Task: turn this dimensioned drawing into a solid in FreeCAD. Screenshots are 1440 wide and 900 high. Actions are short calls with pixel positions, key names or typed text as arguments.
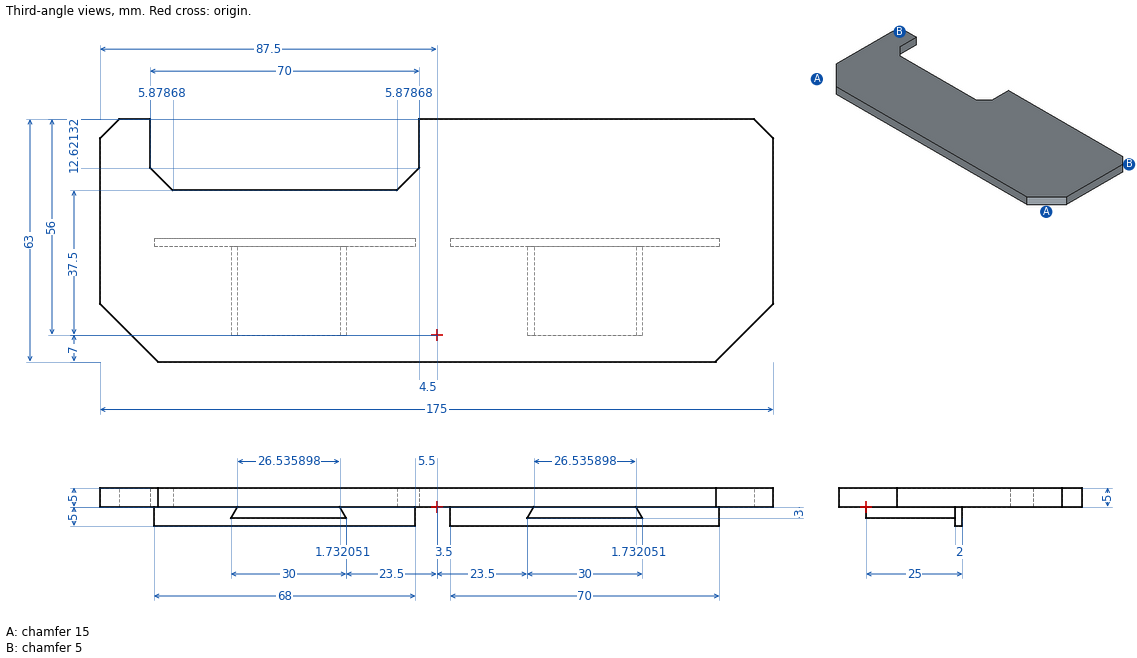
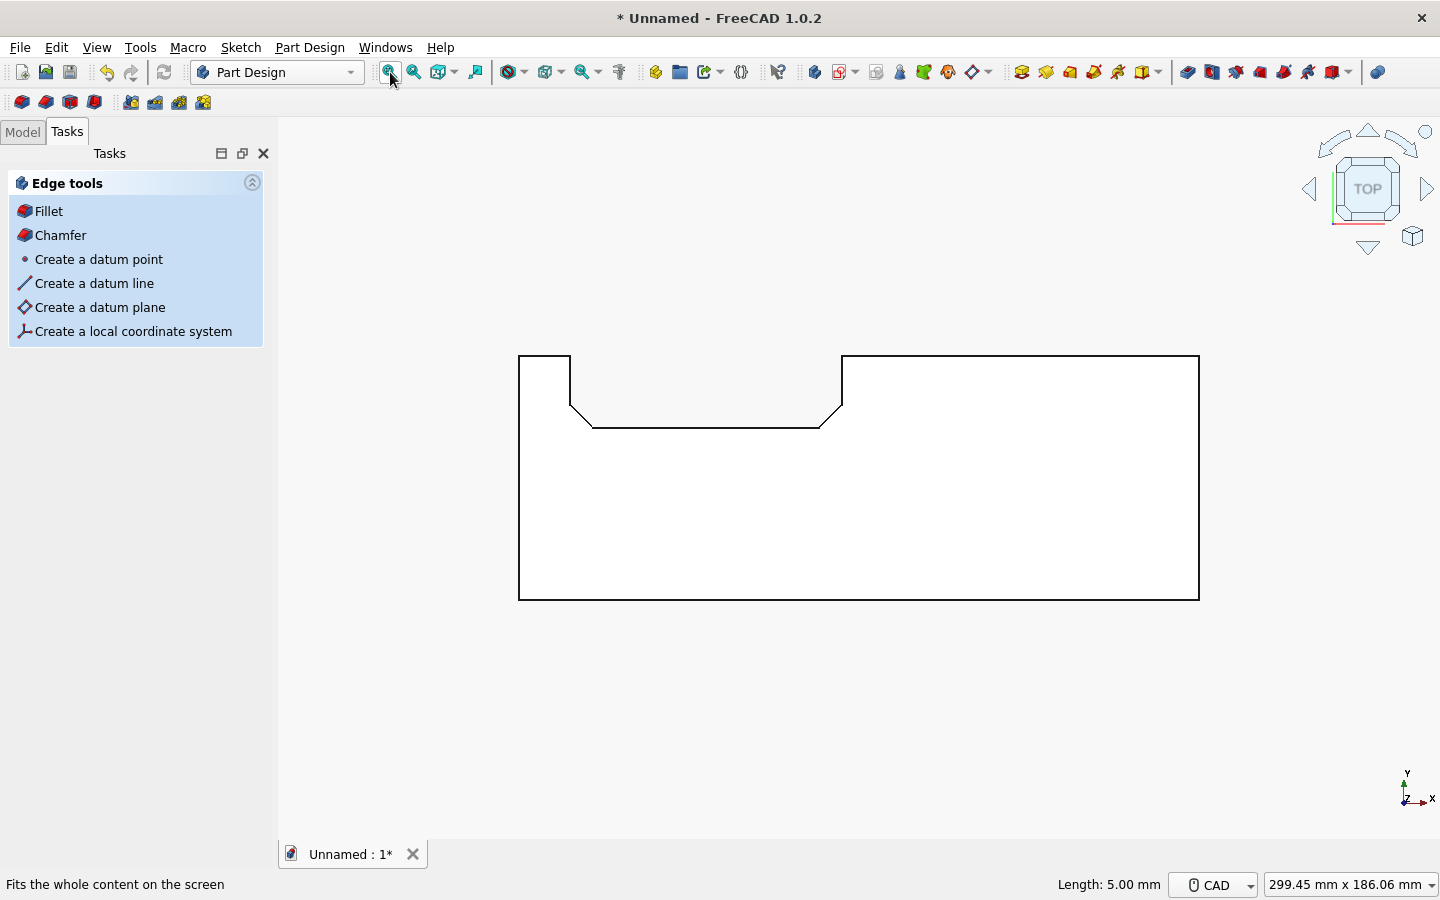
scroll(519, 599, up, 4)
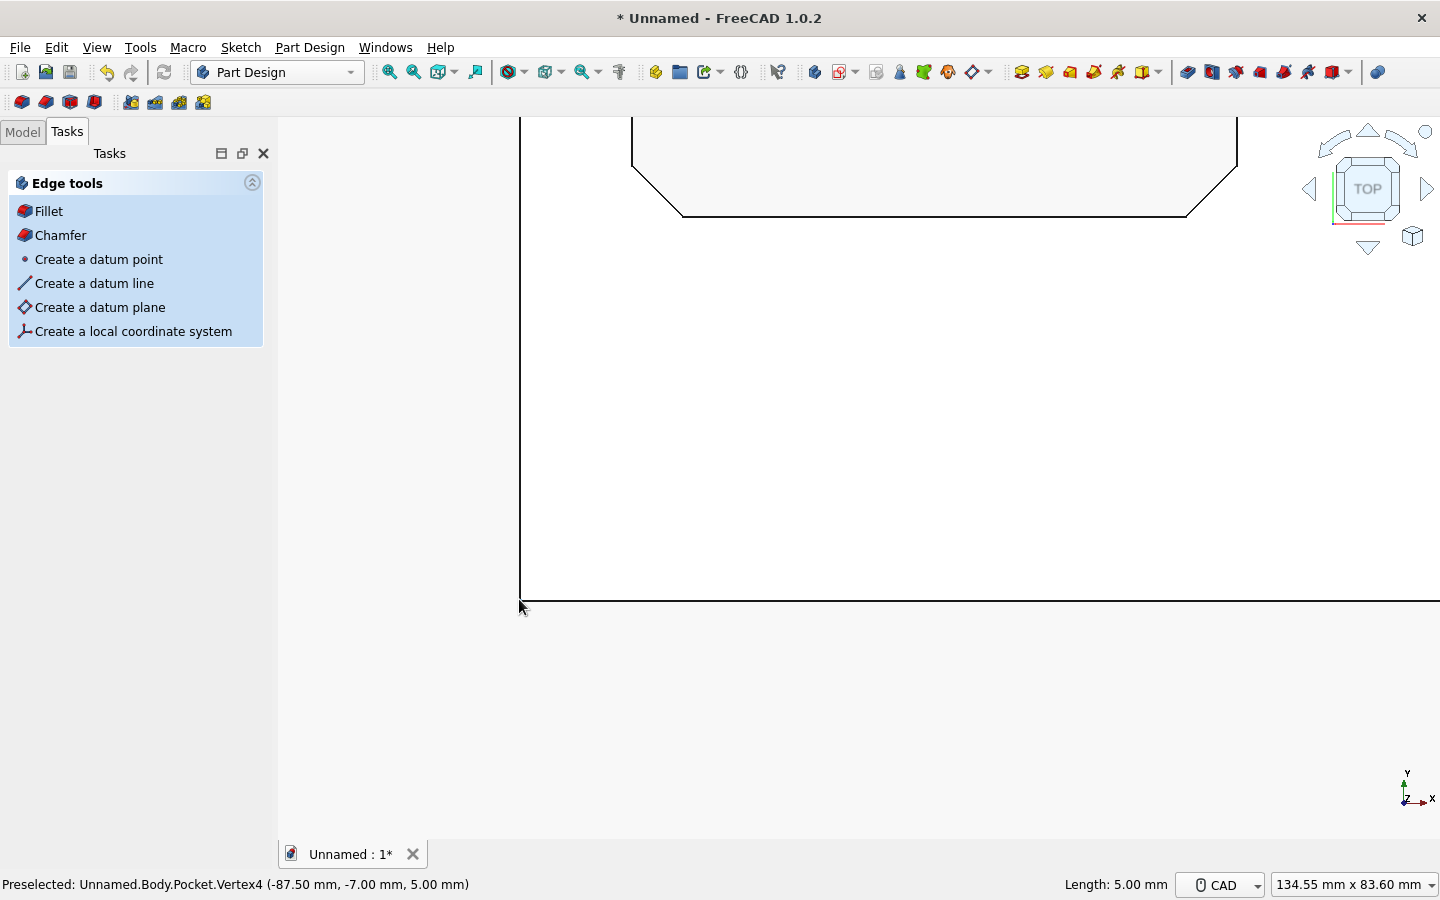
key(v)
key(f)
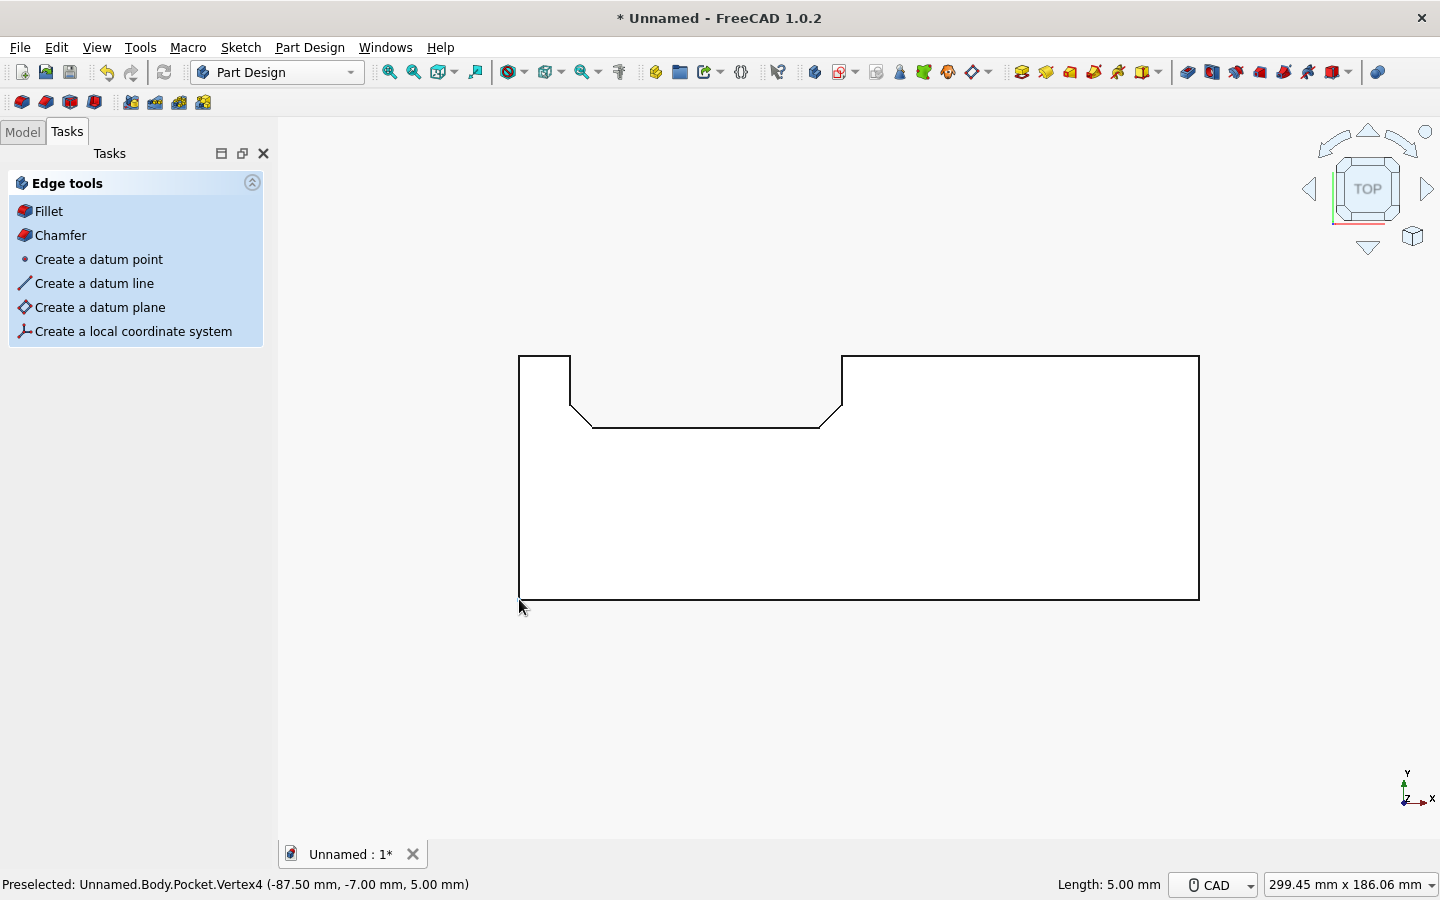
key(1)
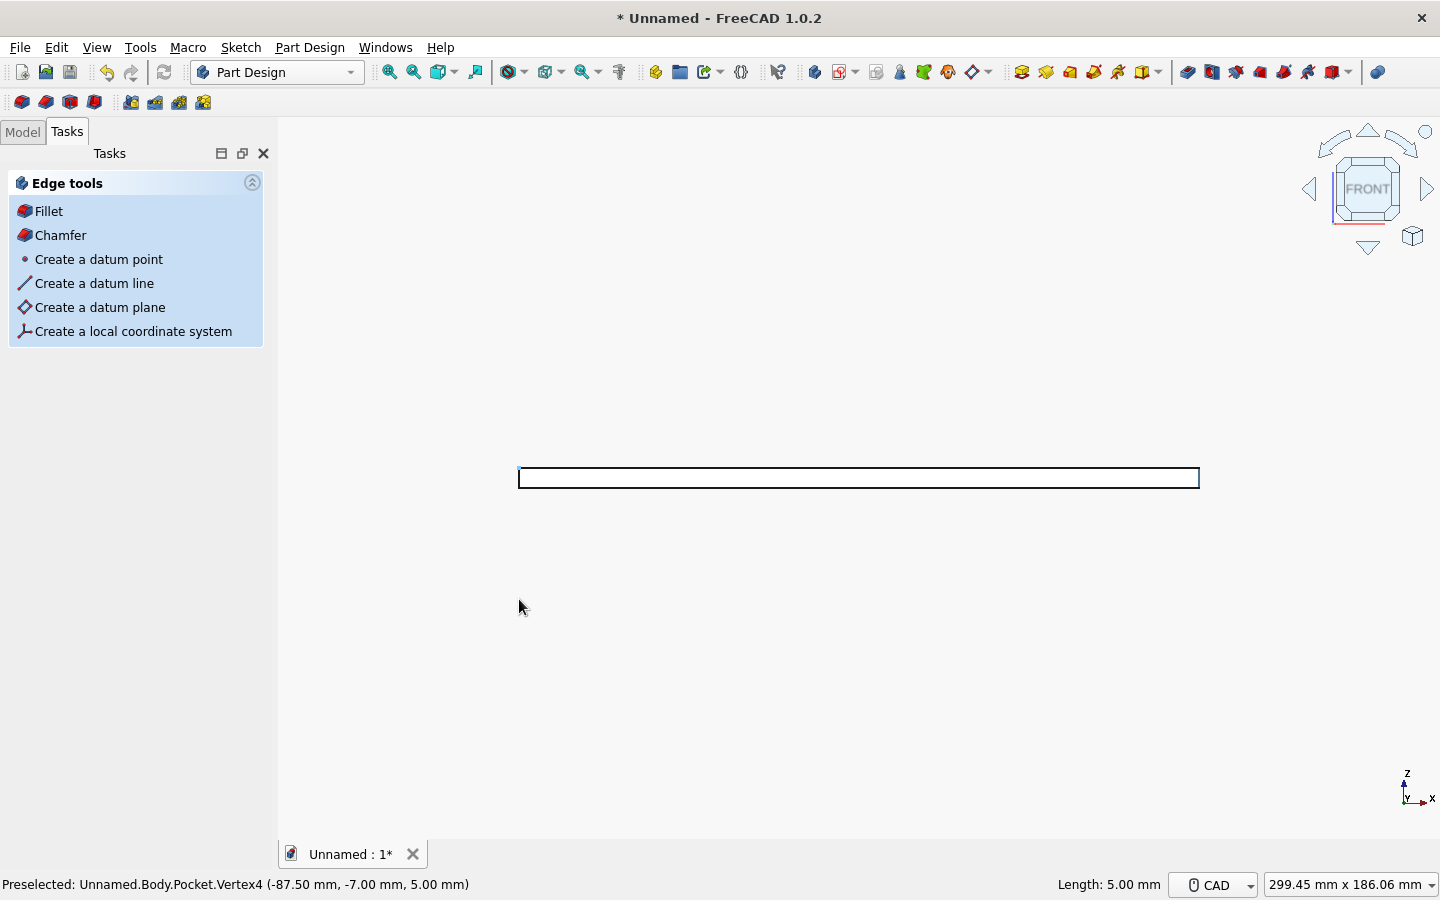
click(519, 477, ctrl)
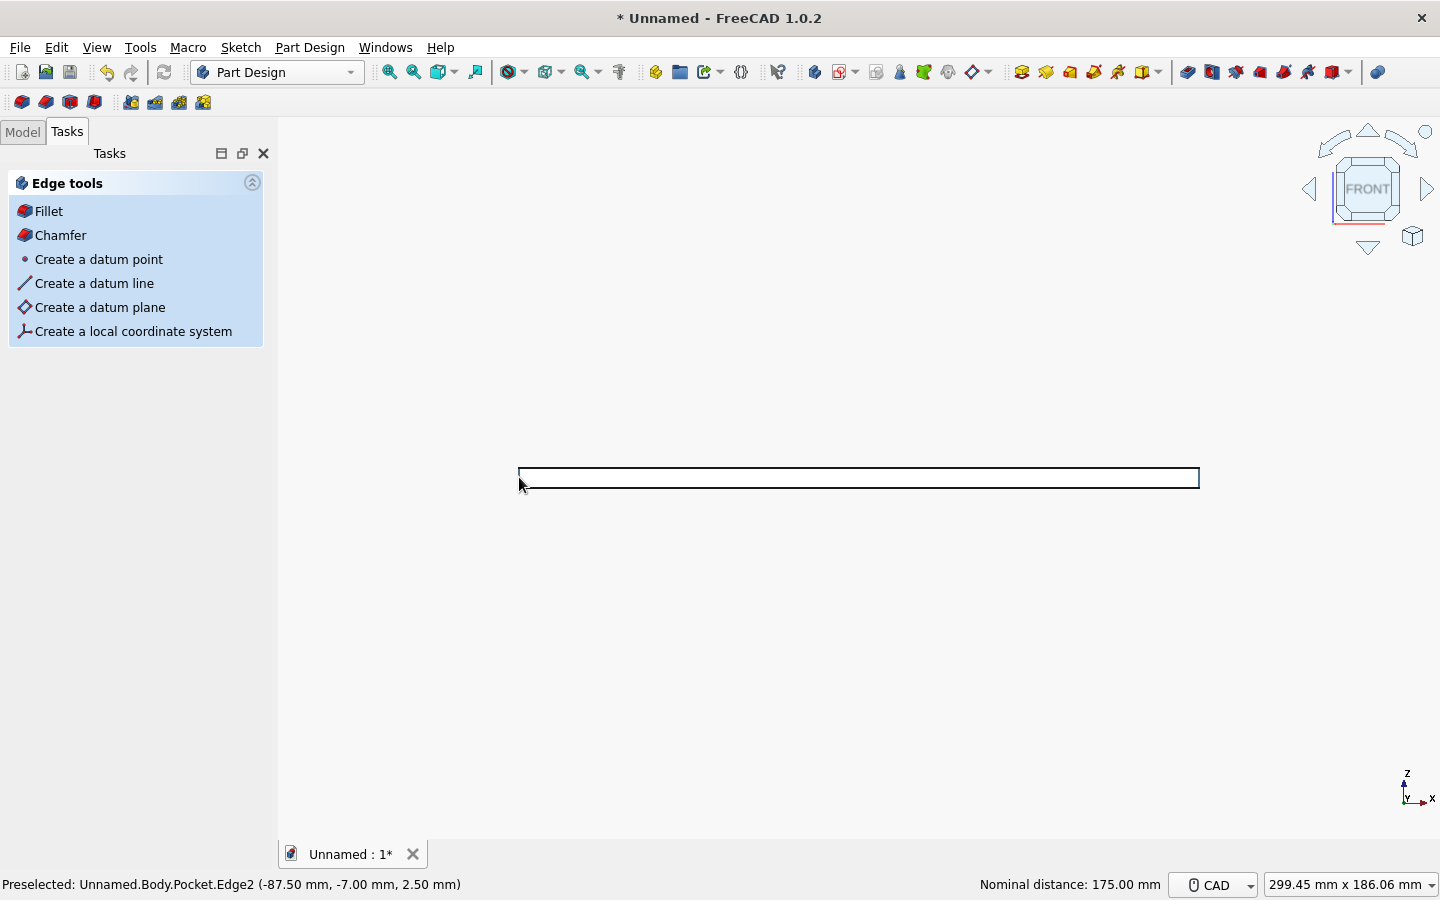
click(46, 102)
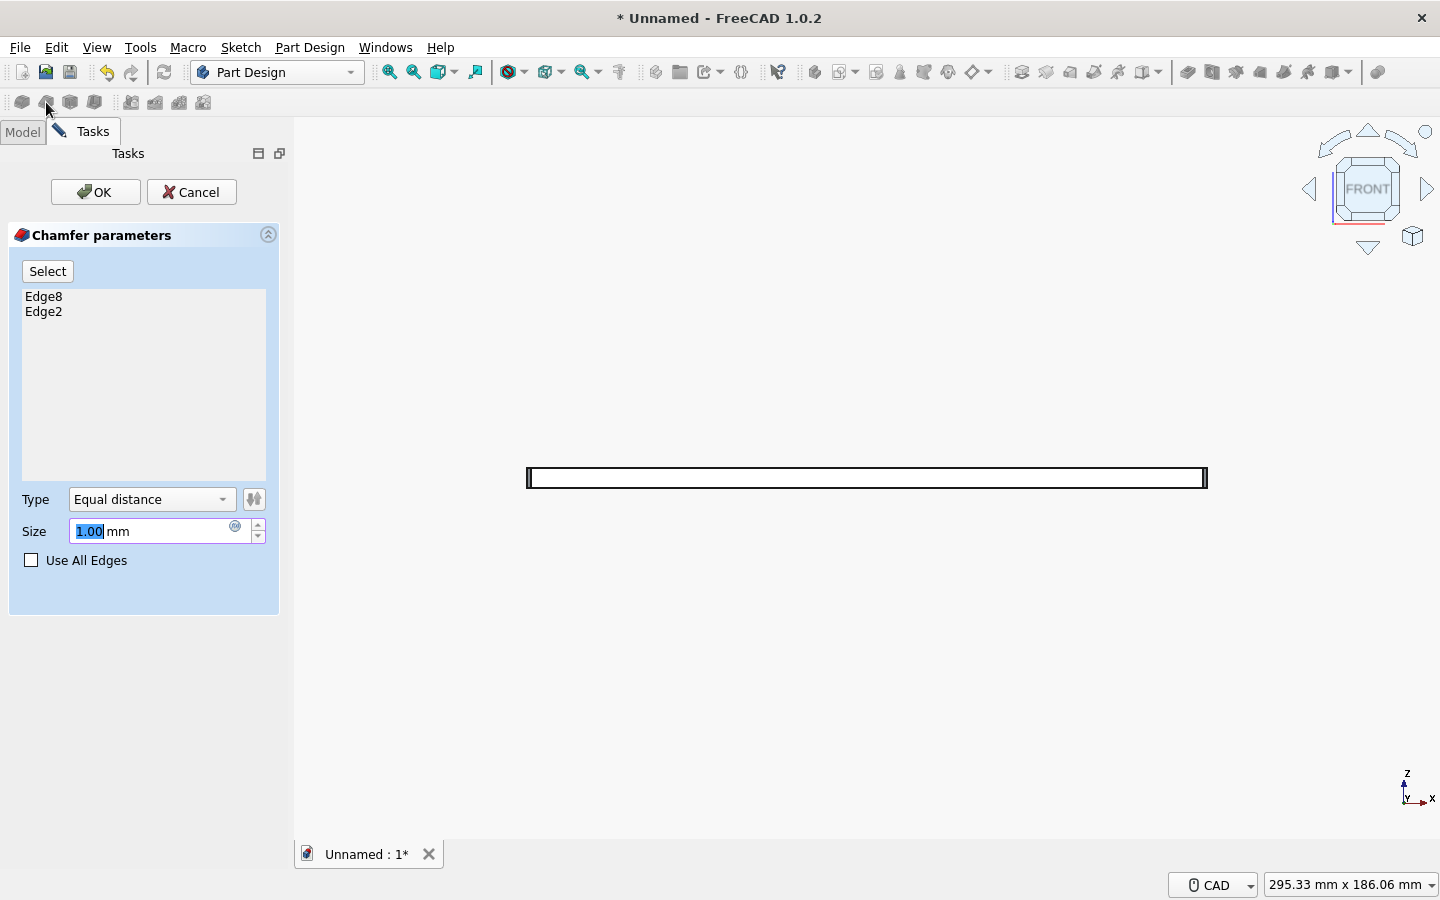
text(15)
key(Tab)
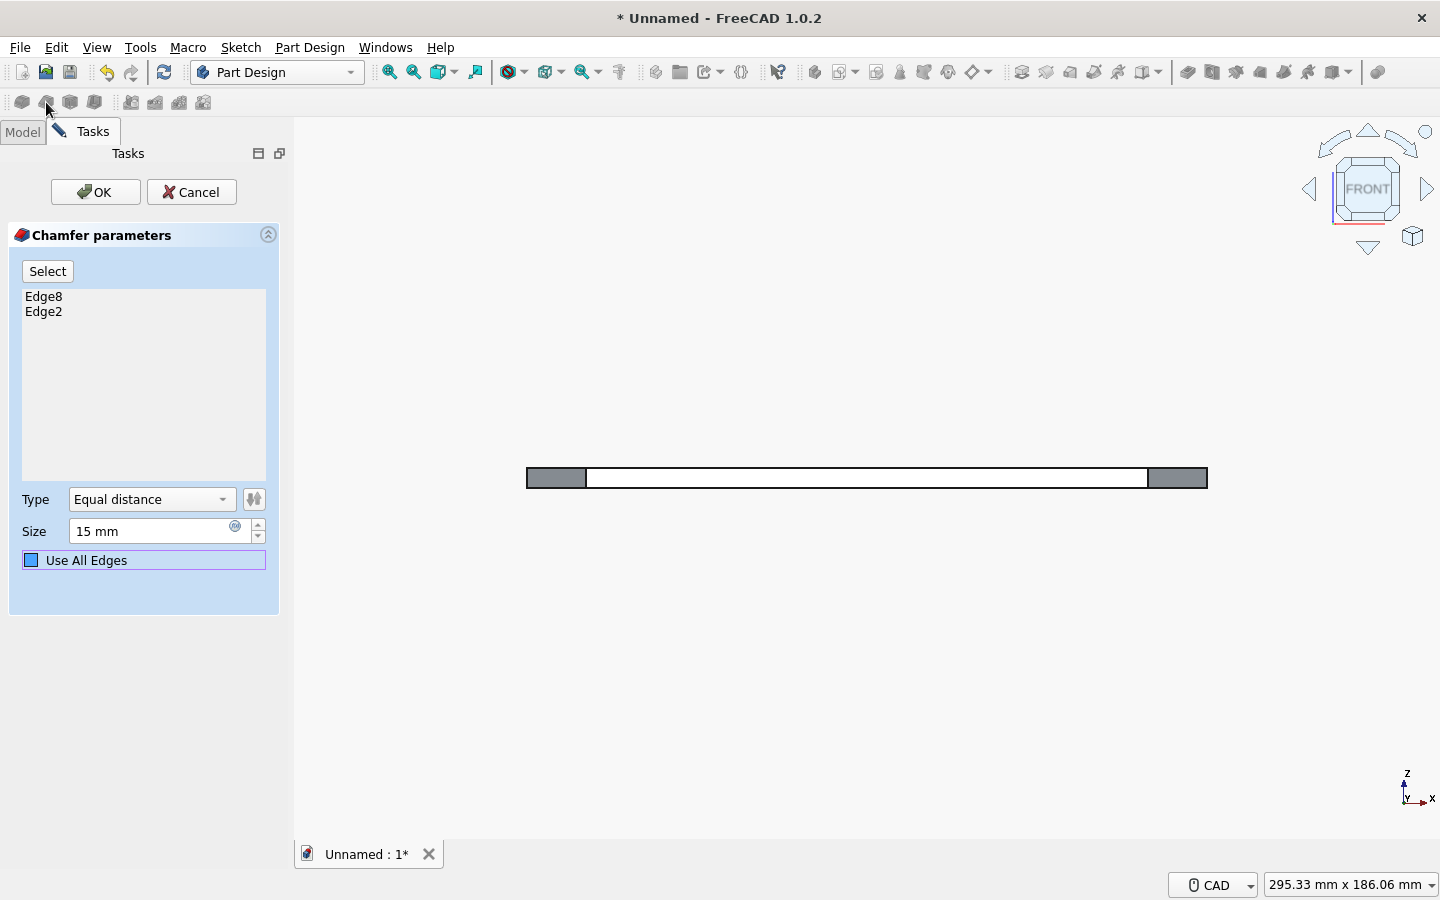
click(96, 192)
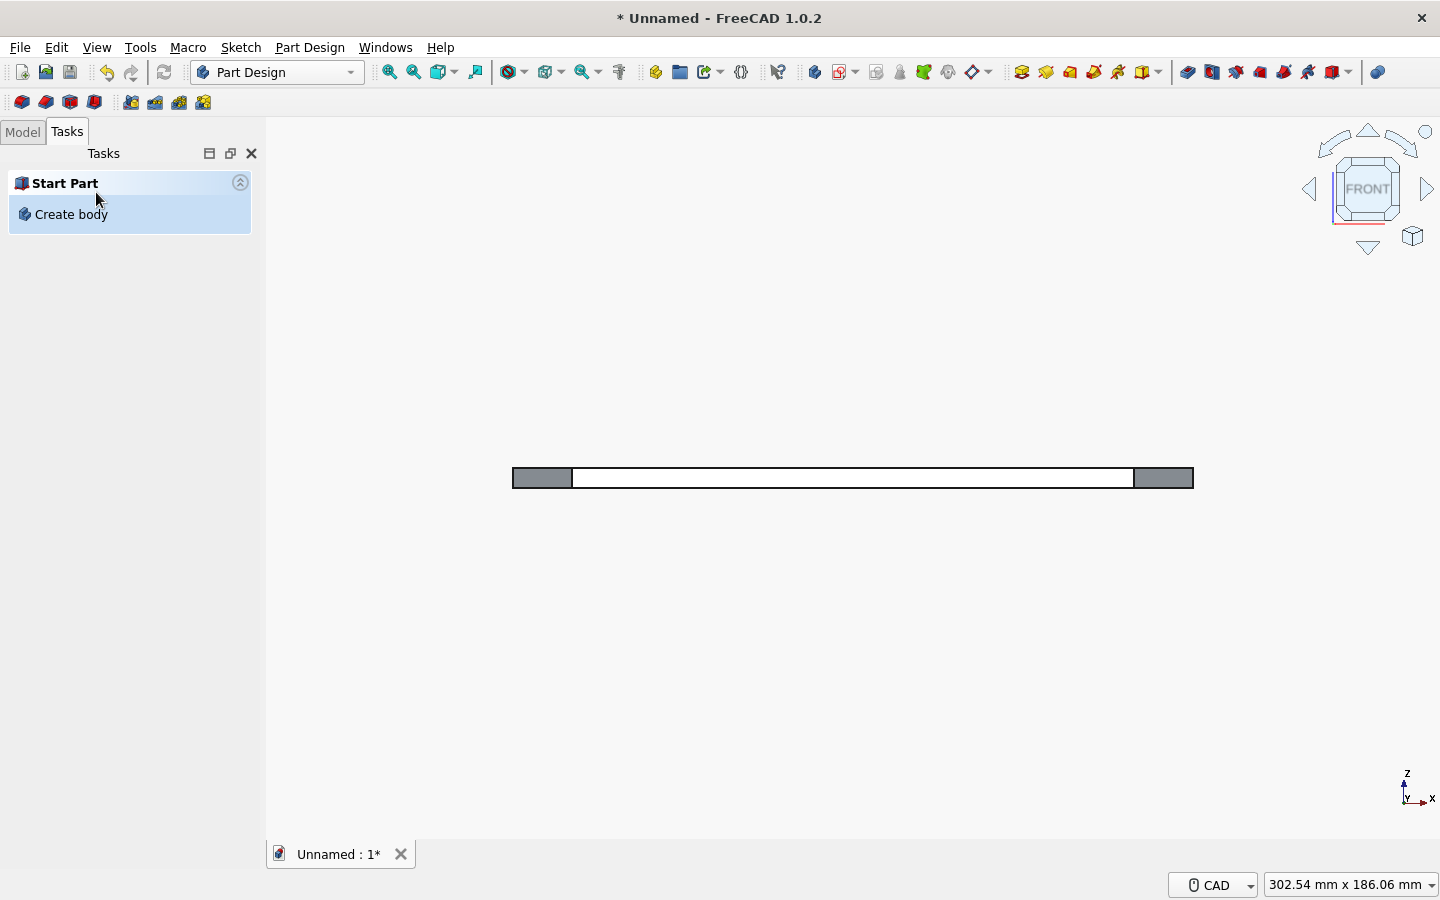
scroll(513, 477, up, 4)